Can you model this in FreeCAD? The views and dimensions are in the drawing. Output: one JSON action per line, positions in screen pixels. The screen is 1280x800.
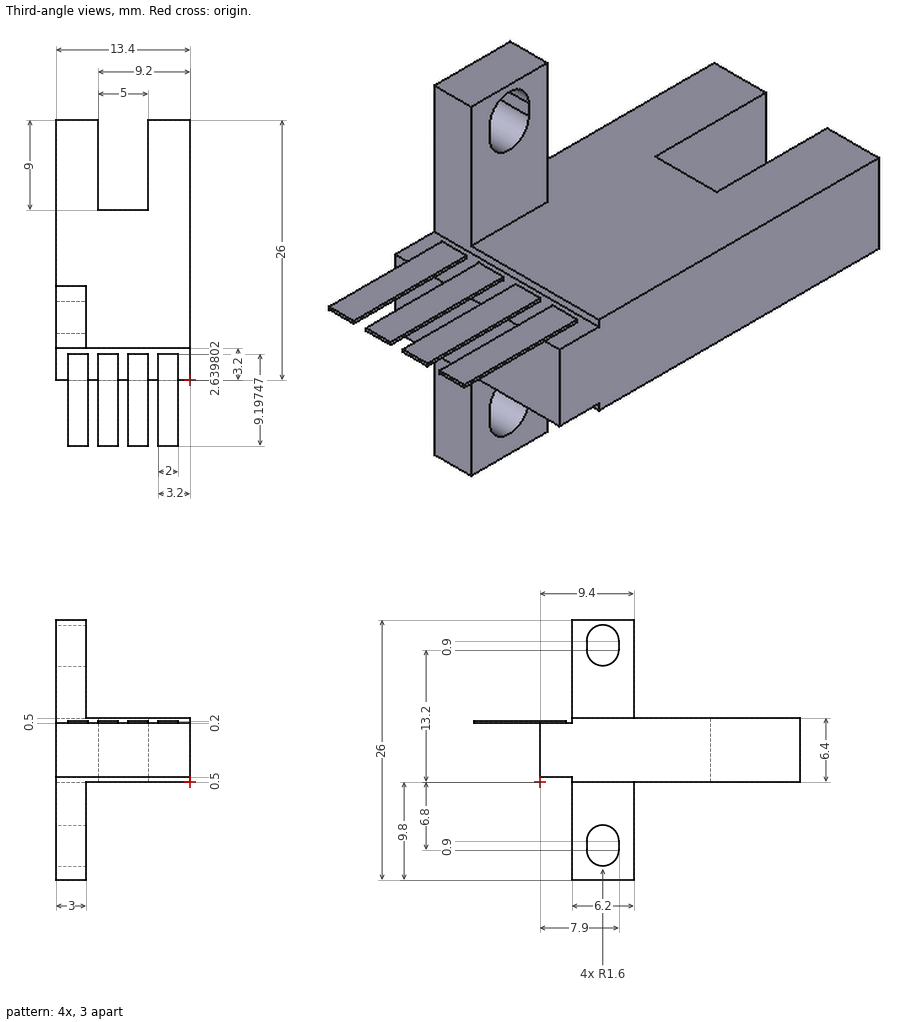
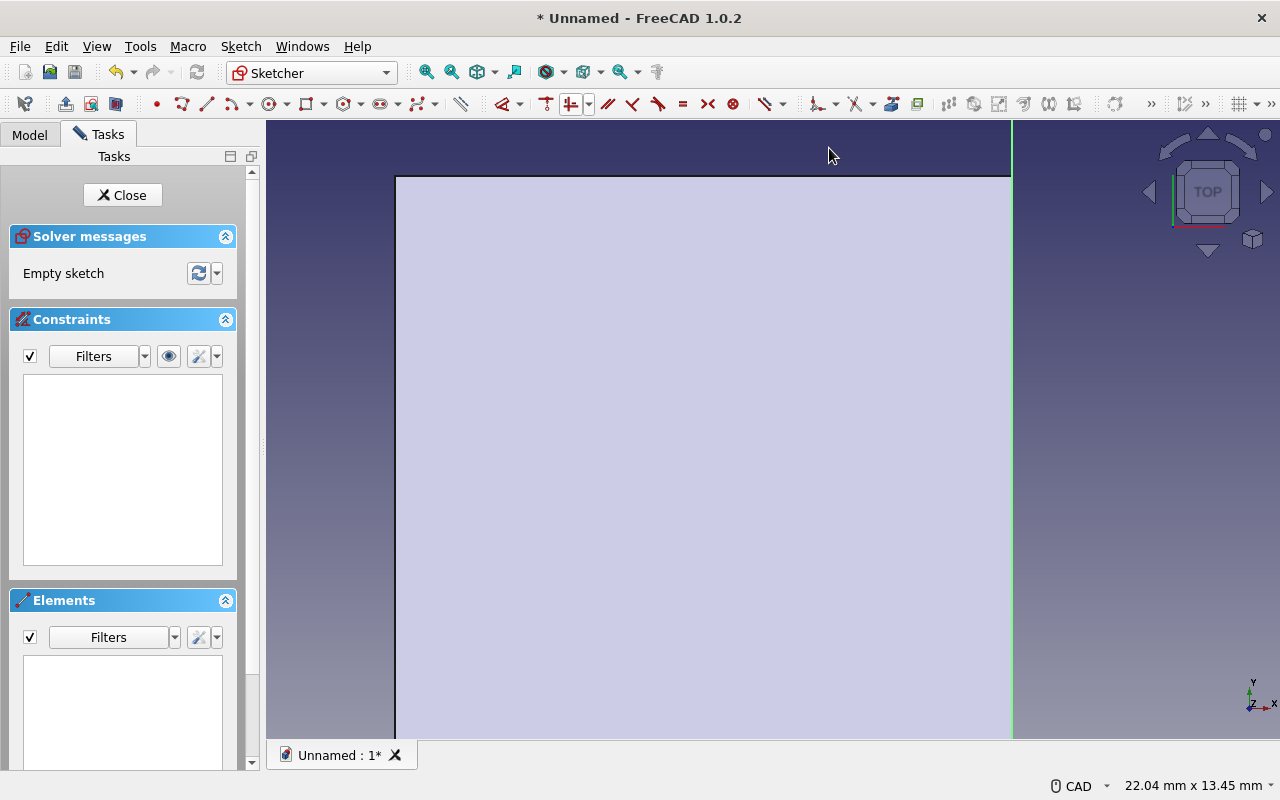
{"action": "key", "text": "g r"}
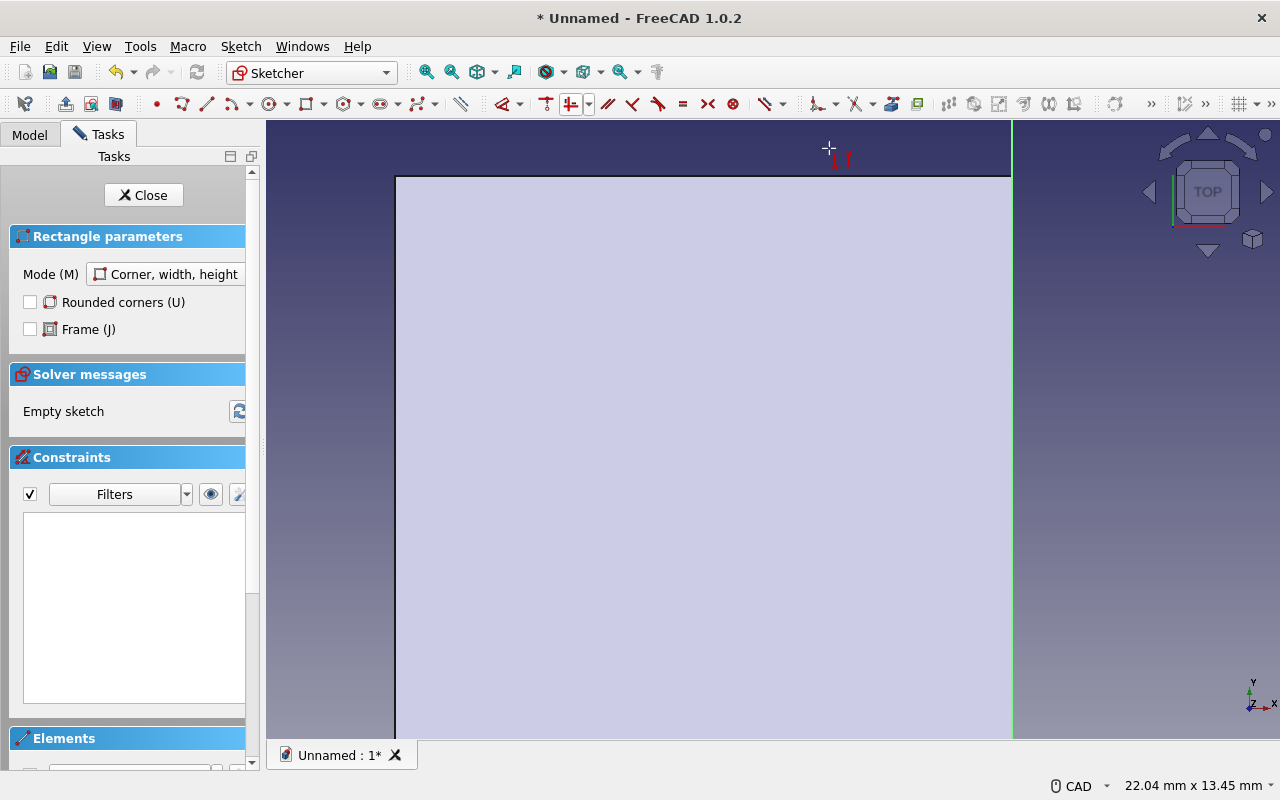
{"action": "left_click", "coordinate": [589, 176]}
{"action": "left_click", "coordinate": [819, 590]}
{"action": "key", "text": "Escape"}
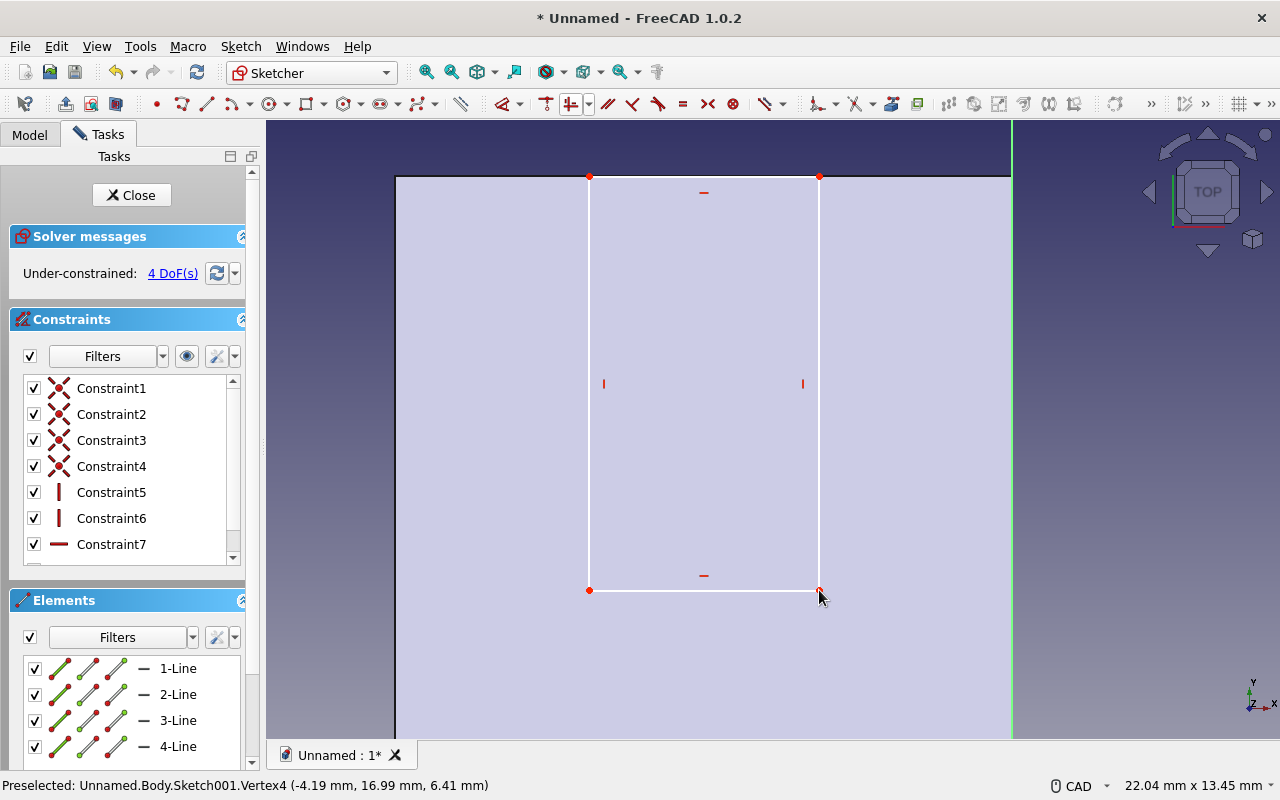
{"action": "key", "text": "d"}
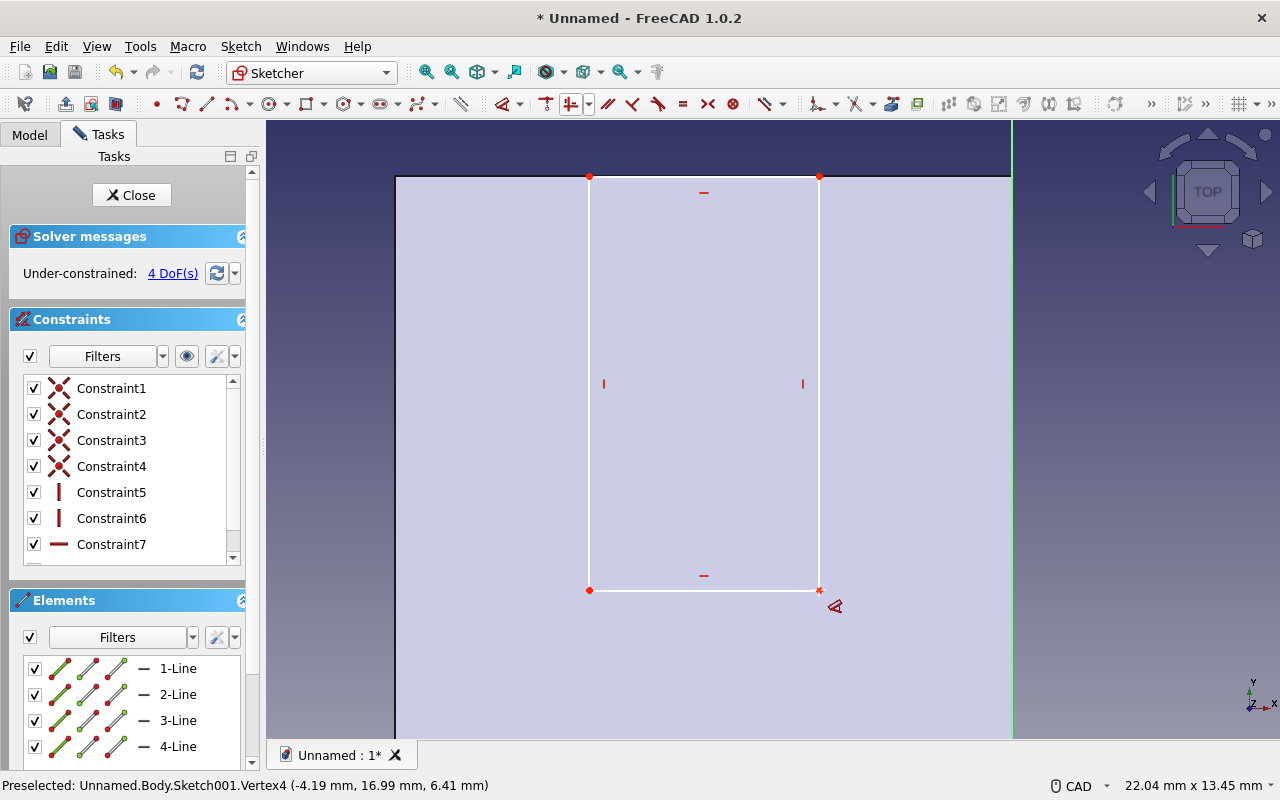
{"action": "left_click", "coordinate": [589, 301]}
{"action": "left_click", "coordinate": [555, 384]}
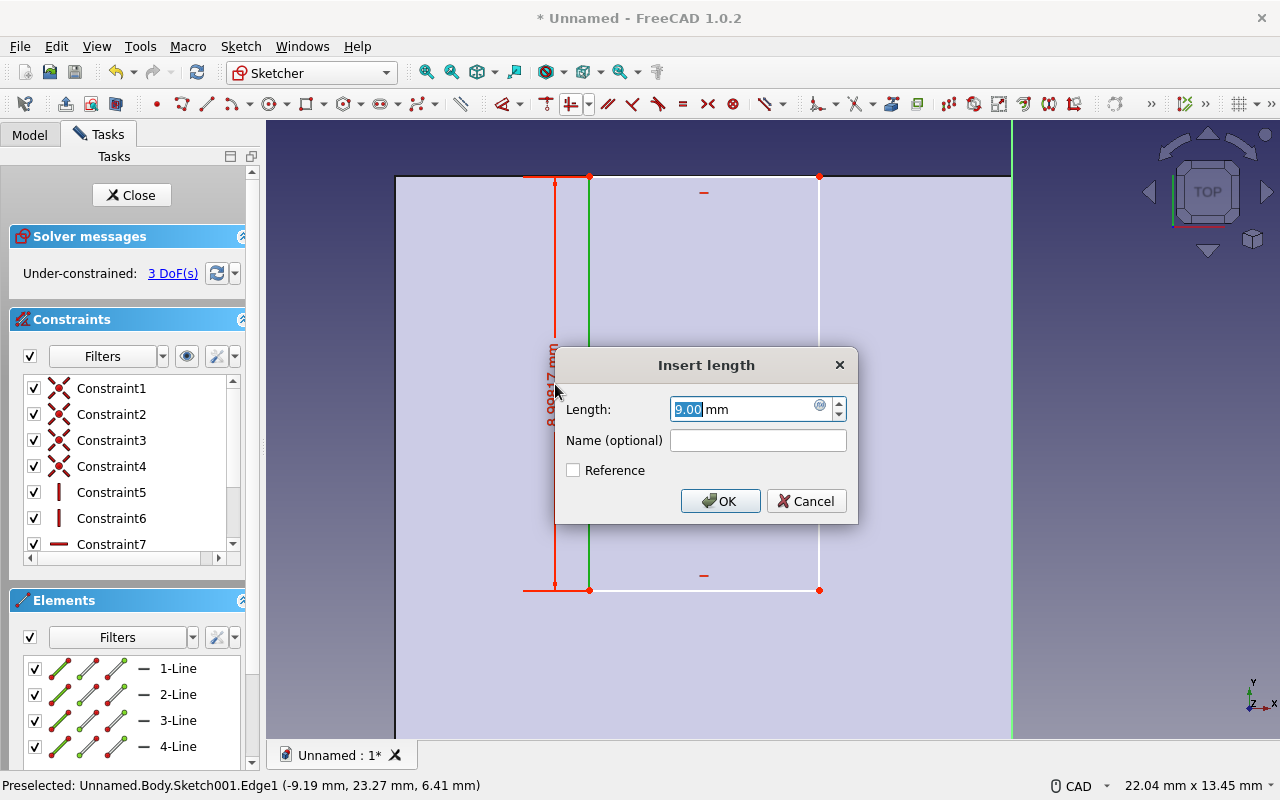
{"action": "type", "text": "9"}
{"action": "key", "text": "Return"}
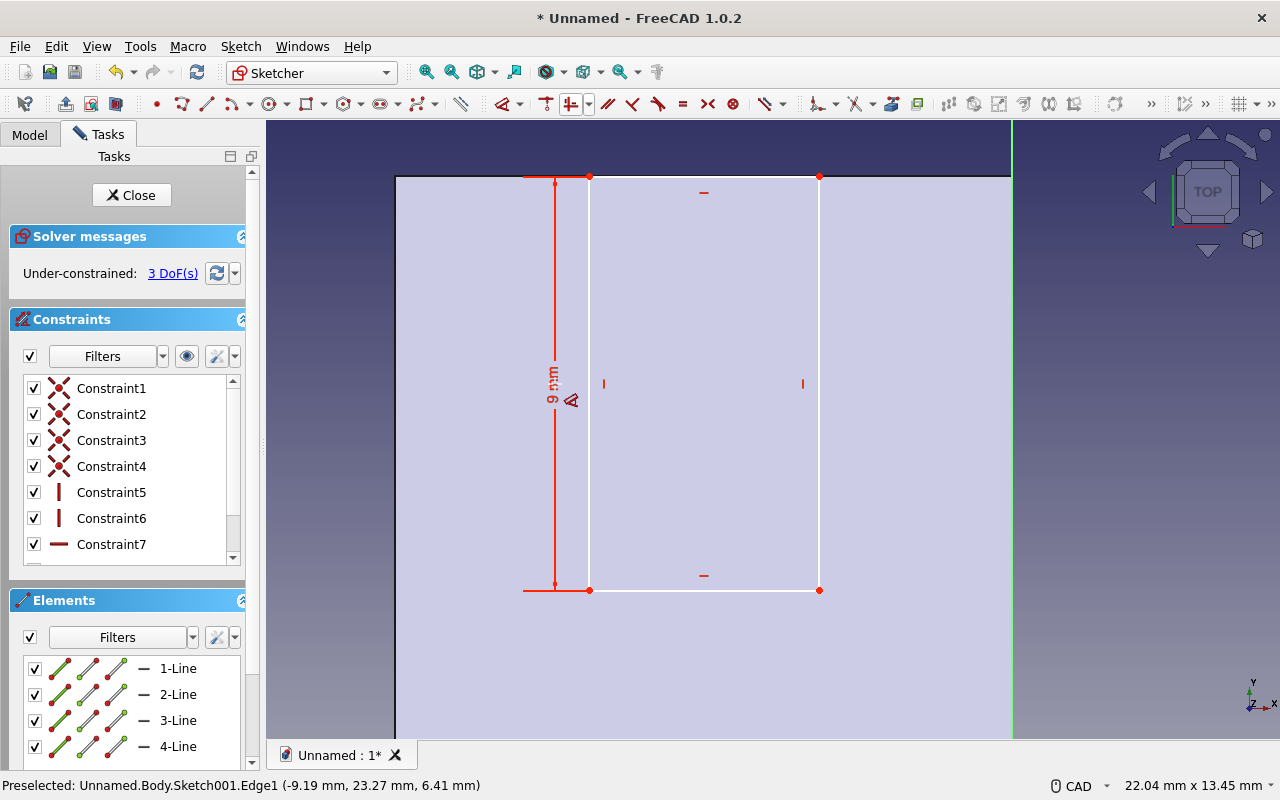
{"action": "left_click", "coordinate": [658, 591]}
{"action": "left_click", "coordinate": [704, 625]}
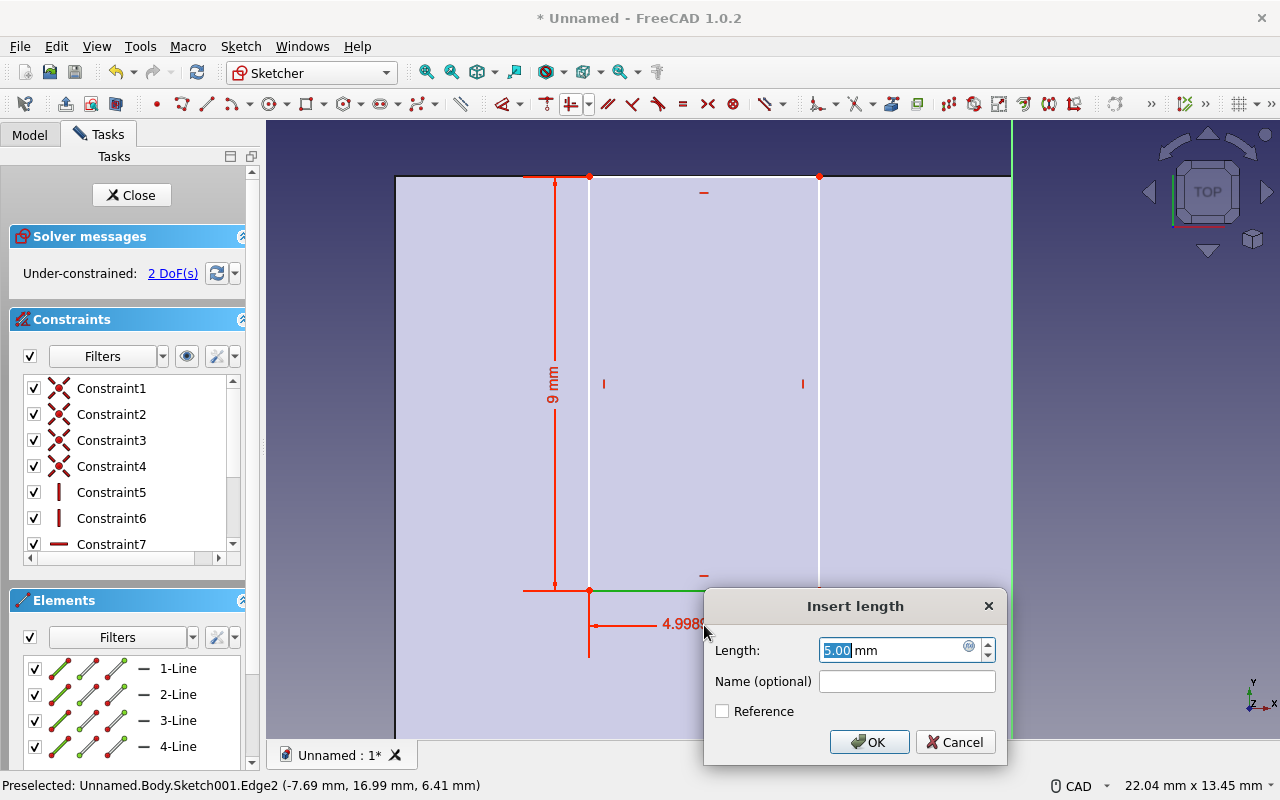
{"action": "type", "text": "5"}
{"action": "key", "text": "Return"}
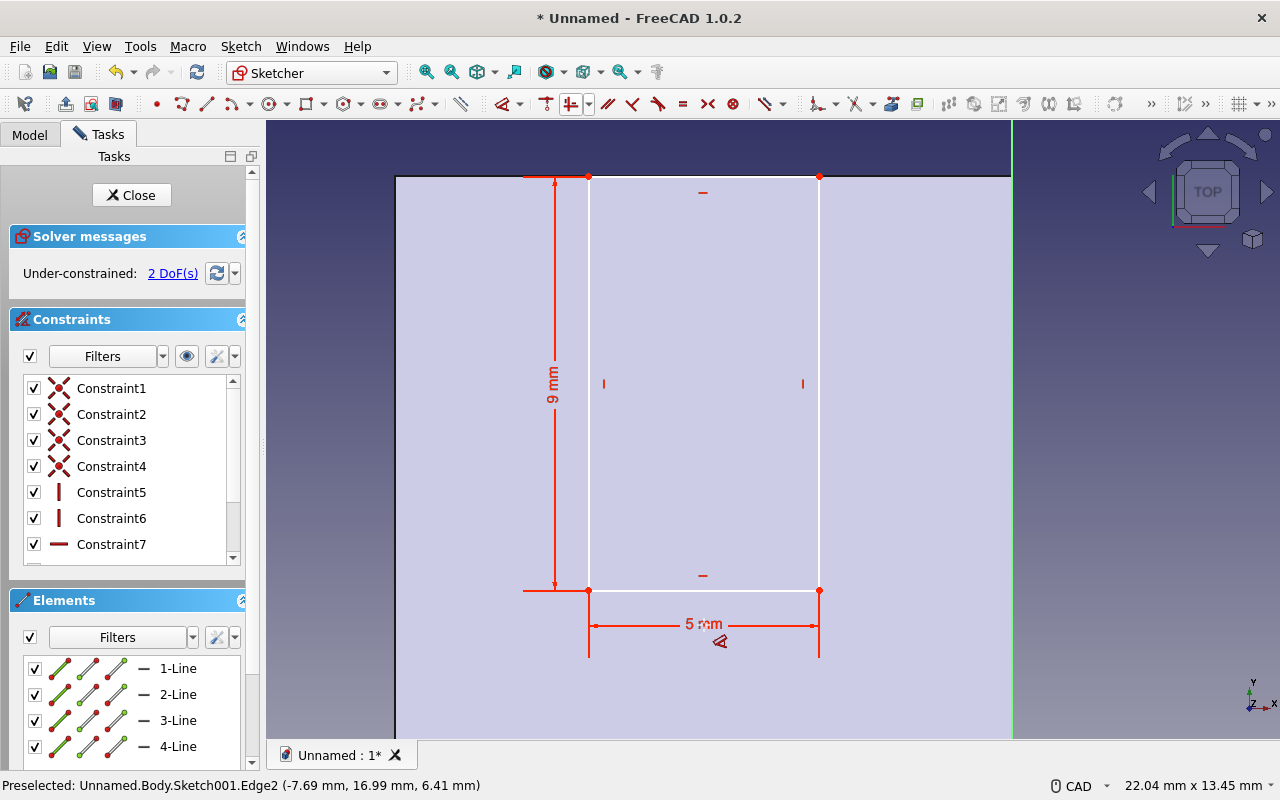
{"action": "left_click", "coordinate": [589, 177]}
{"action": "left_click", "coordinate": [1046, 444]}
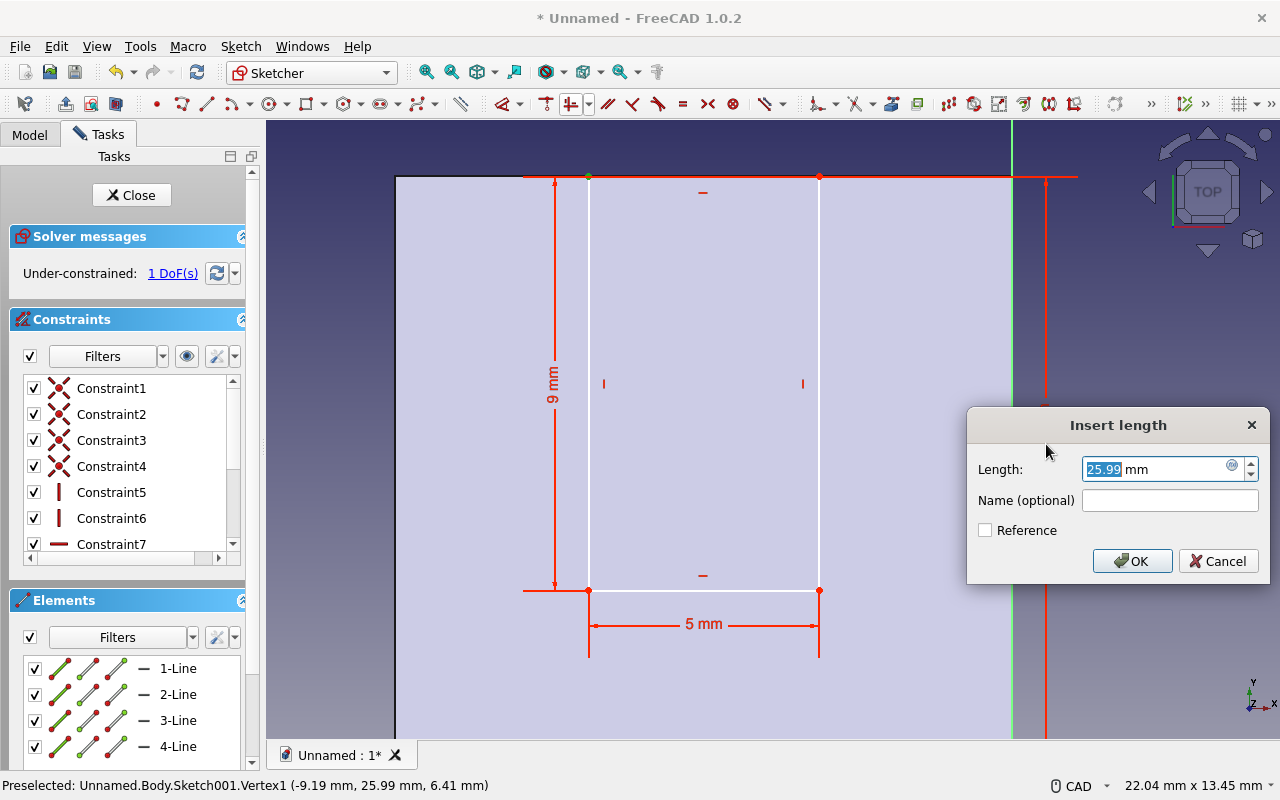
{"action": "type", "text": "26"}
{"action": "key", "text": "Return"}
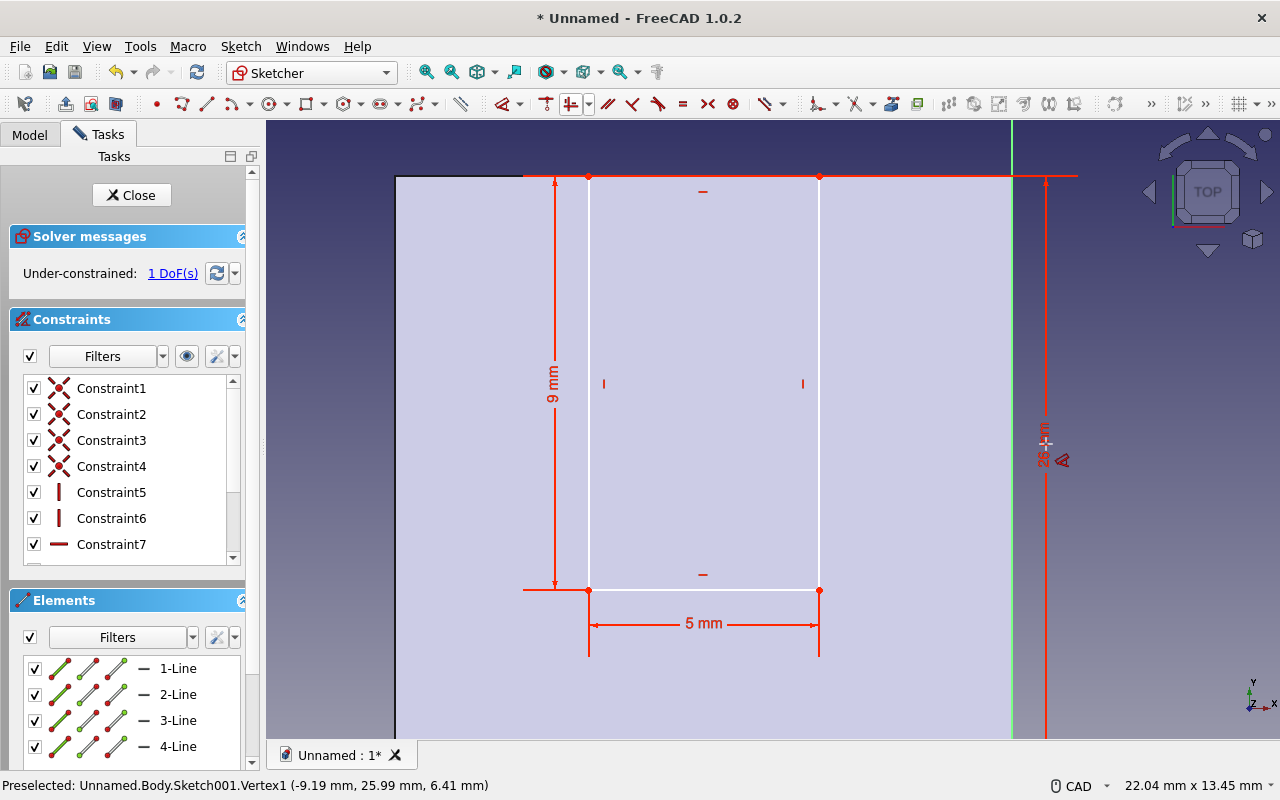
{"action": "left_click", "coordinate": [589, 176]}